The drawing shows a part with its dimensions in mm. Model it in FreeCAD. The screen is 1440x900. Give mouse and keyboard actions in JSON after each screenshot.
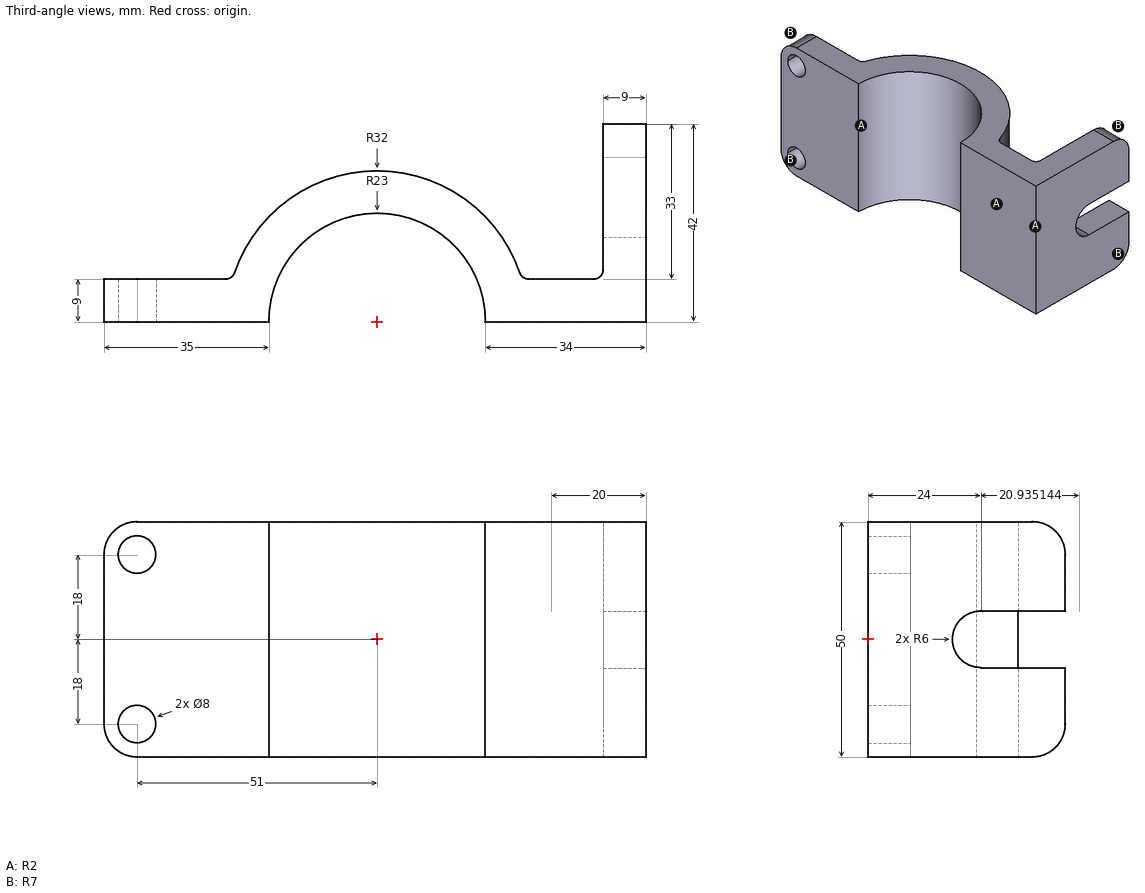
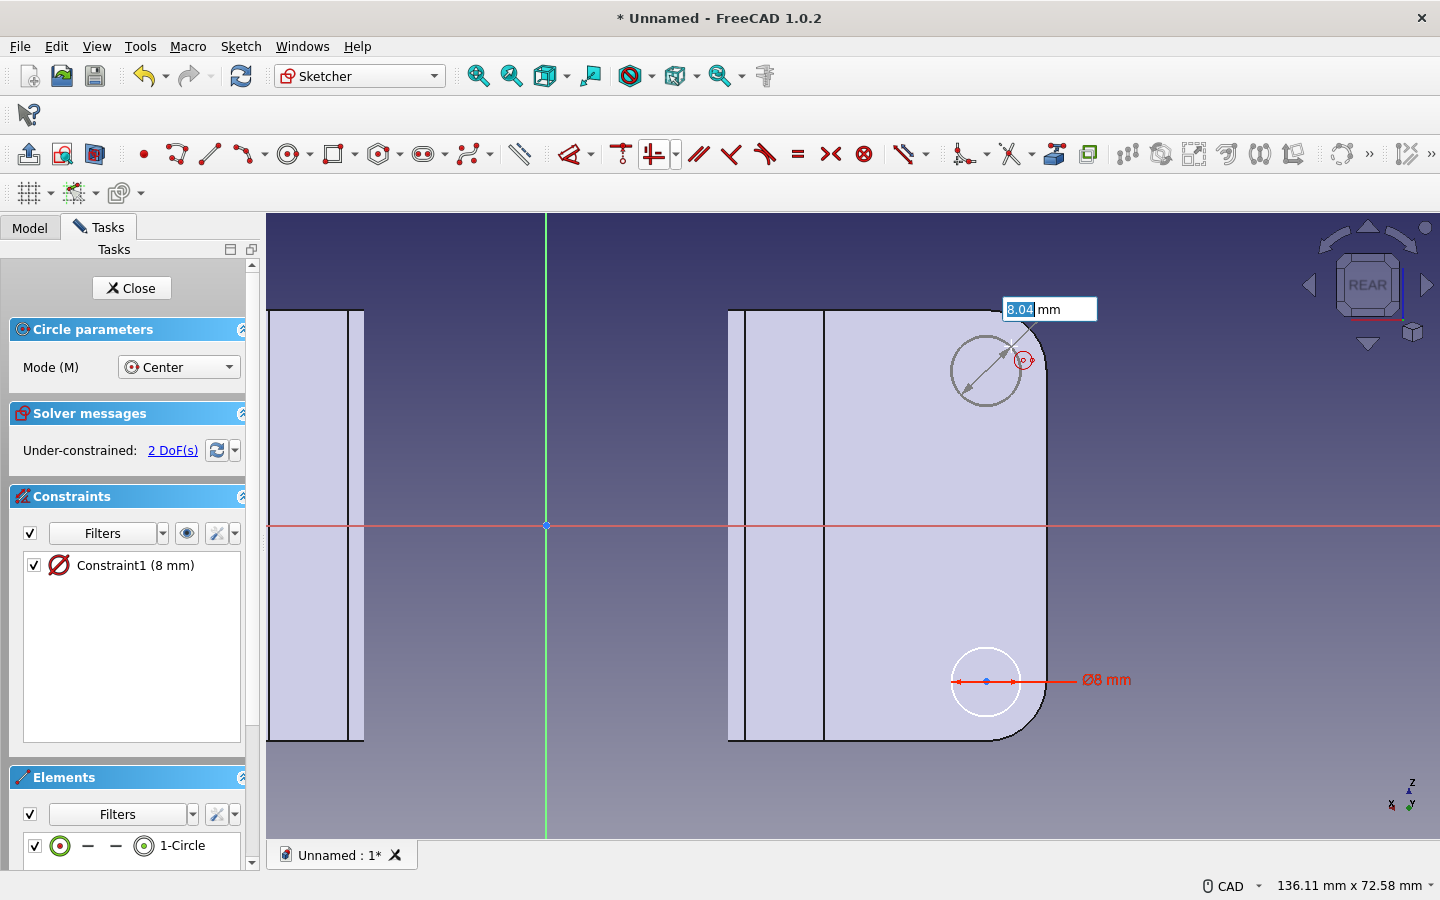
{"action": "type", "text": "8"}
{"action": "key", "text": "Return"}
{"action": "key", "text": "Escape"}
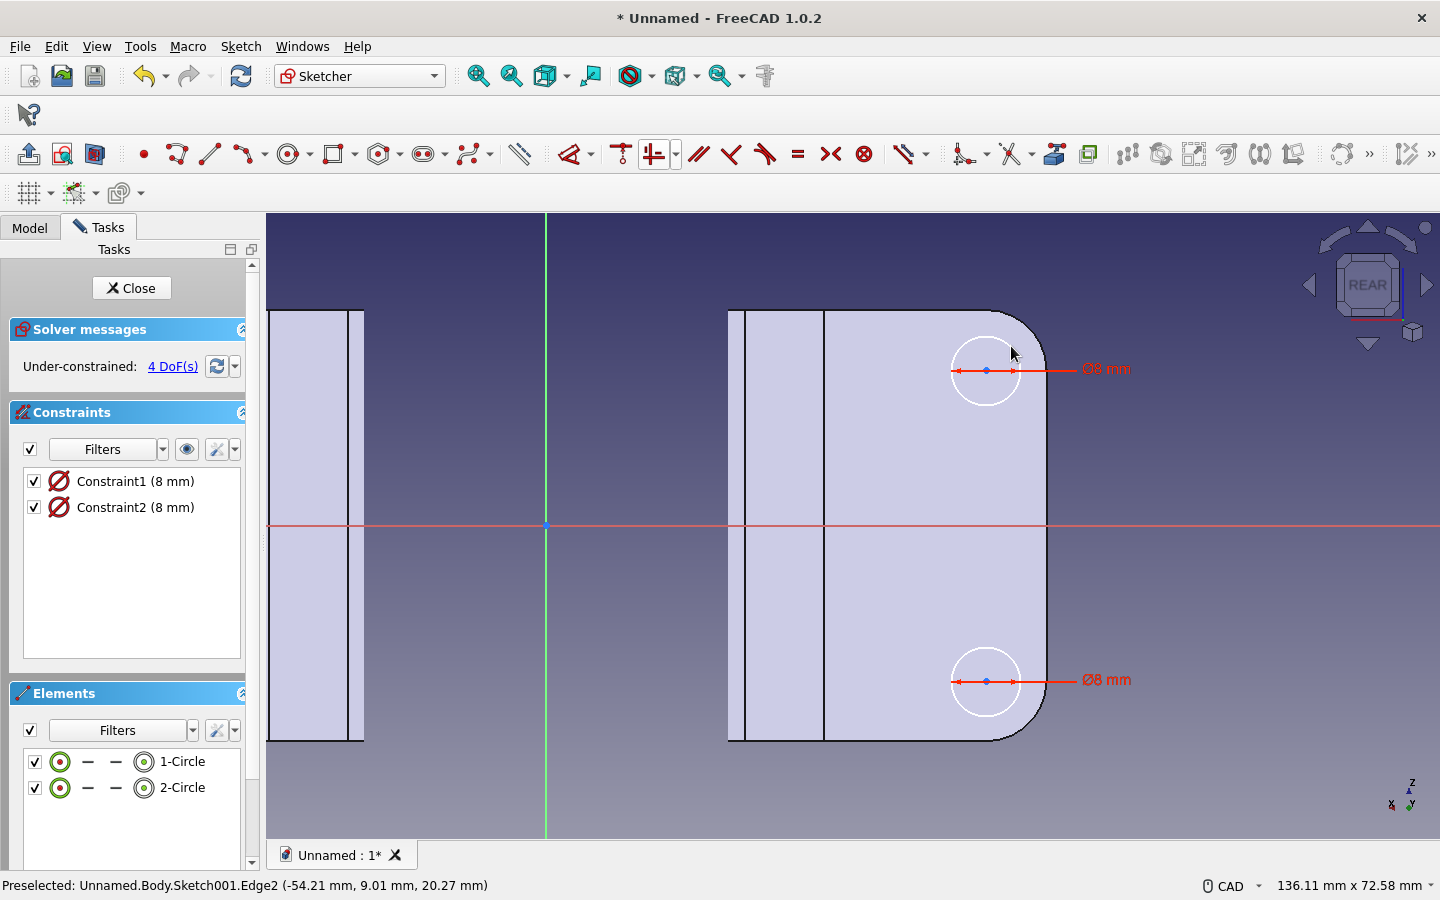
{"action": "left_click", "coordinate": [986, 682]}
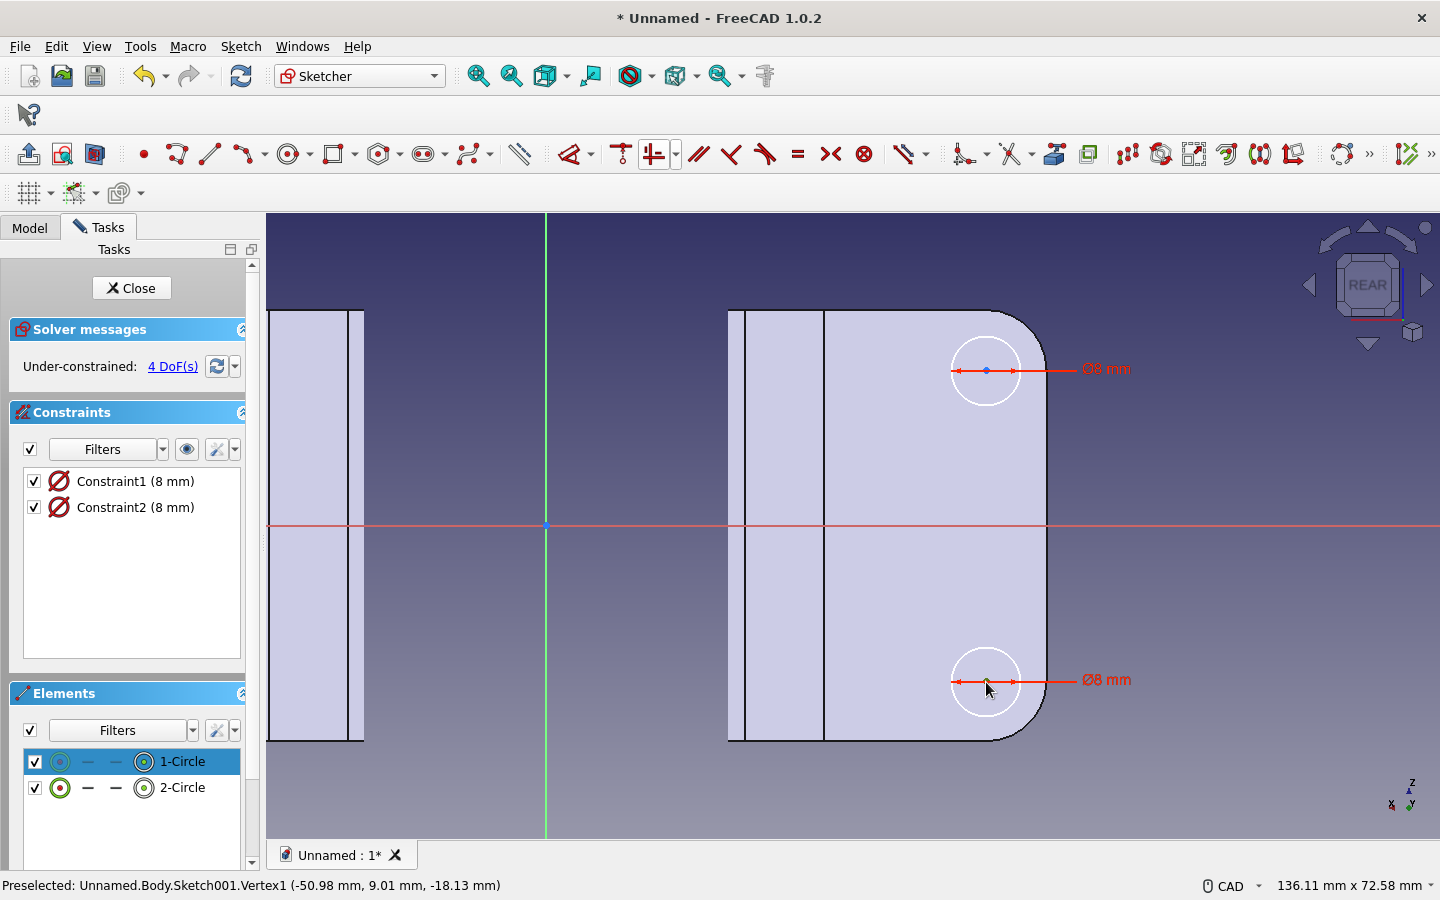
{"action": "left_click", "coordinate": [986, 371]}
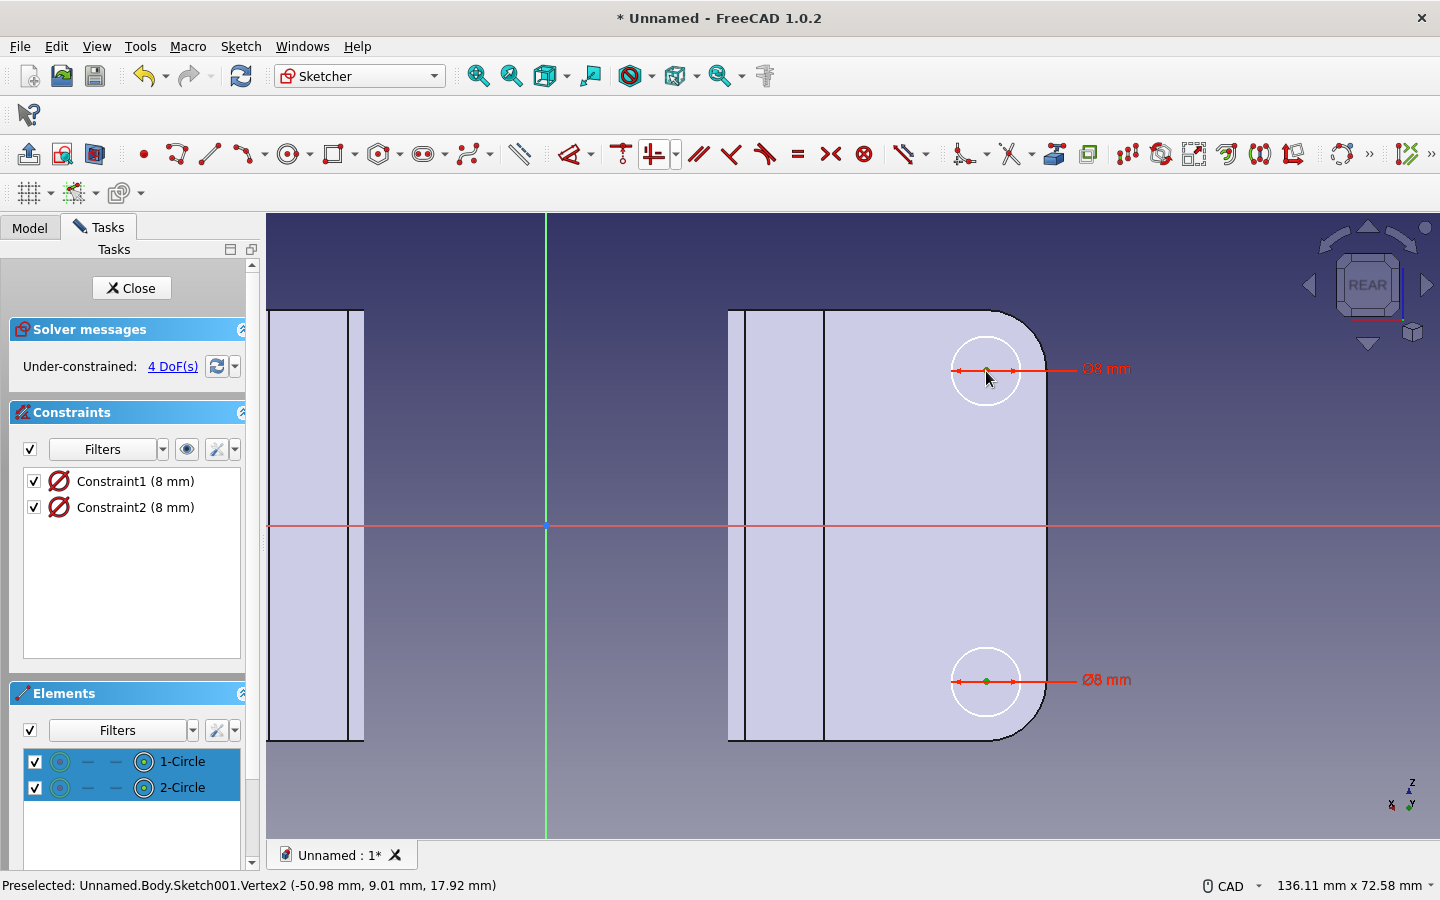
{"action": "key", "text": "v"}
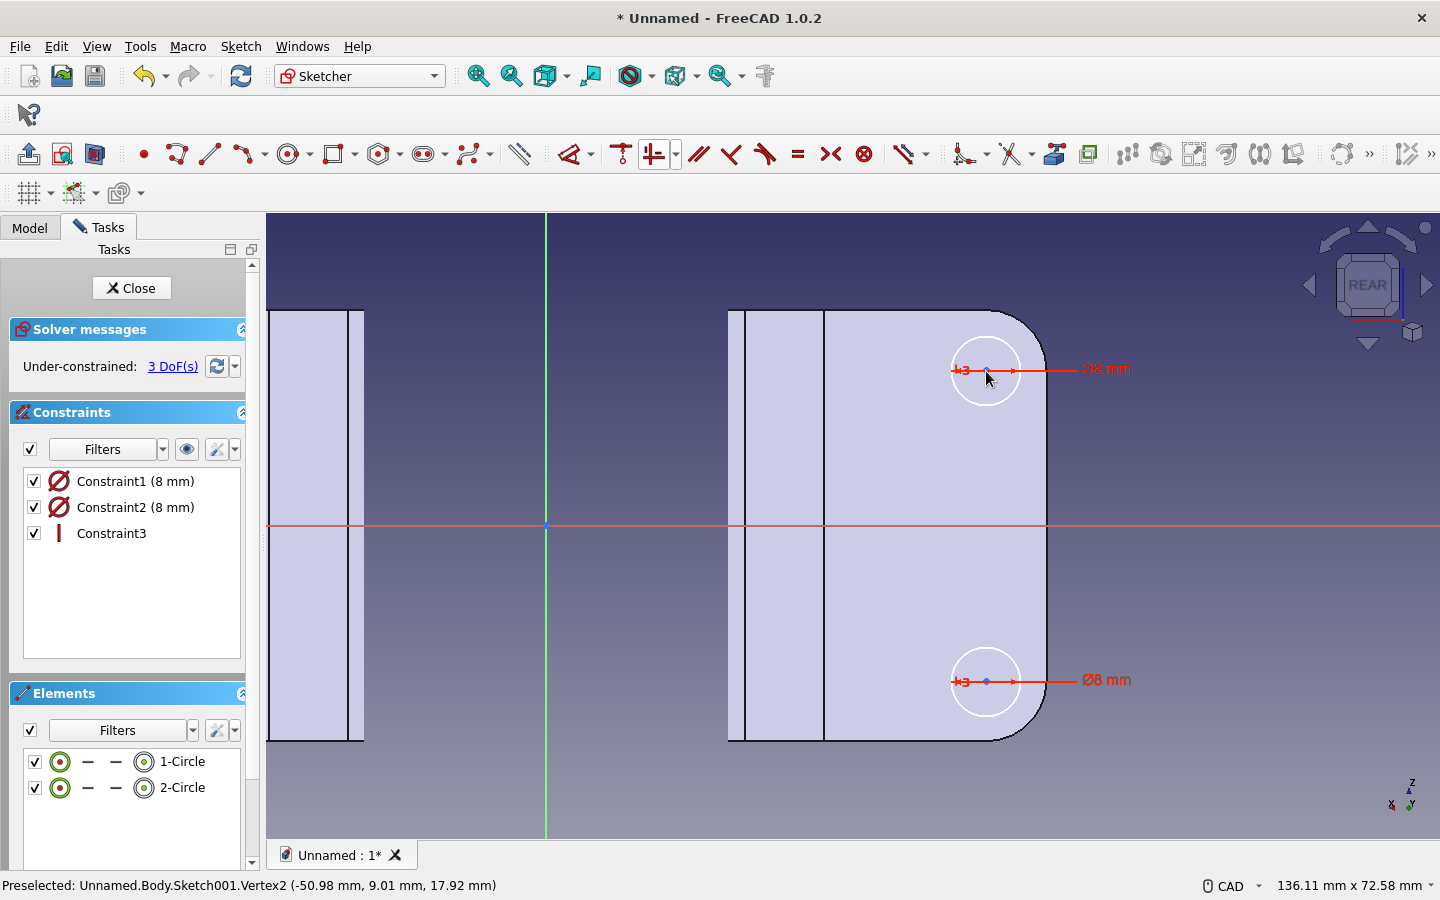
{"action": "left_click", "coordinate": [568, 154]}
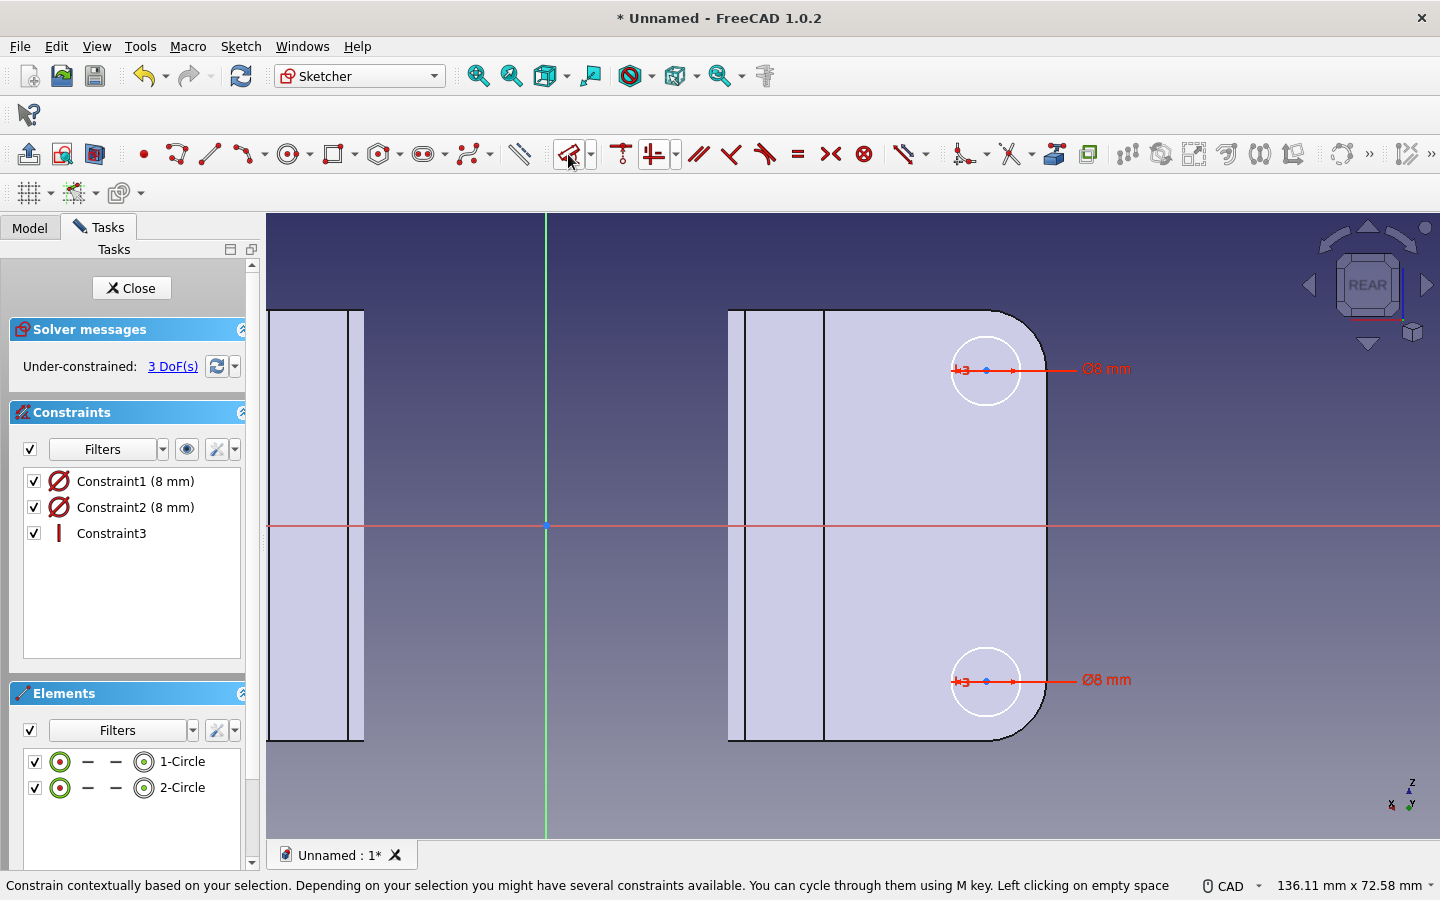
{"action": "left_click", "coordinate": [986, 682]}
{"action": "left_click", "coordinate": [766, 716]}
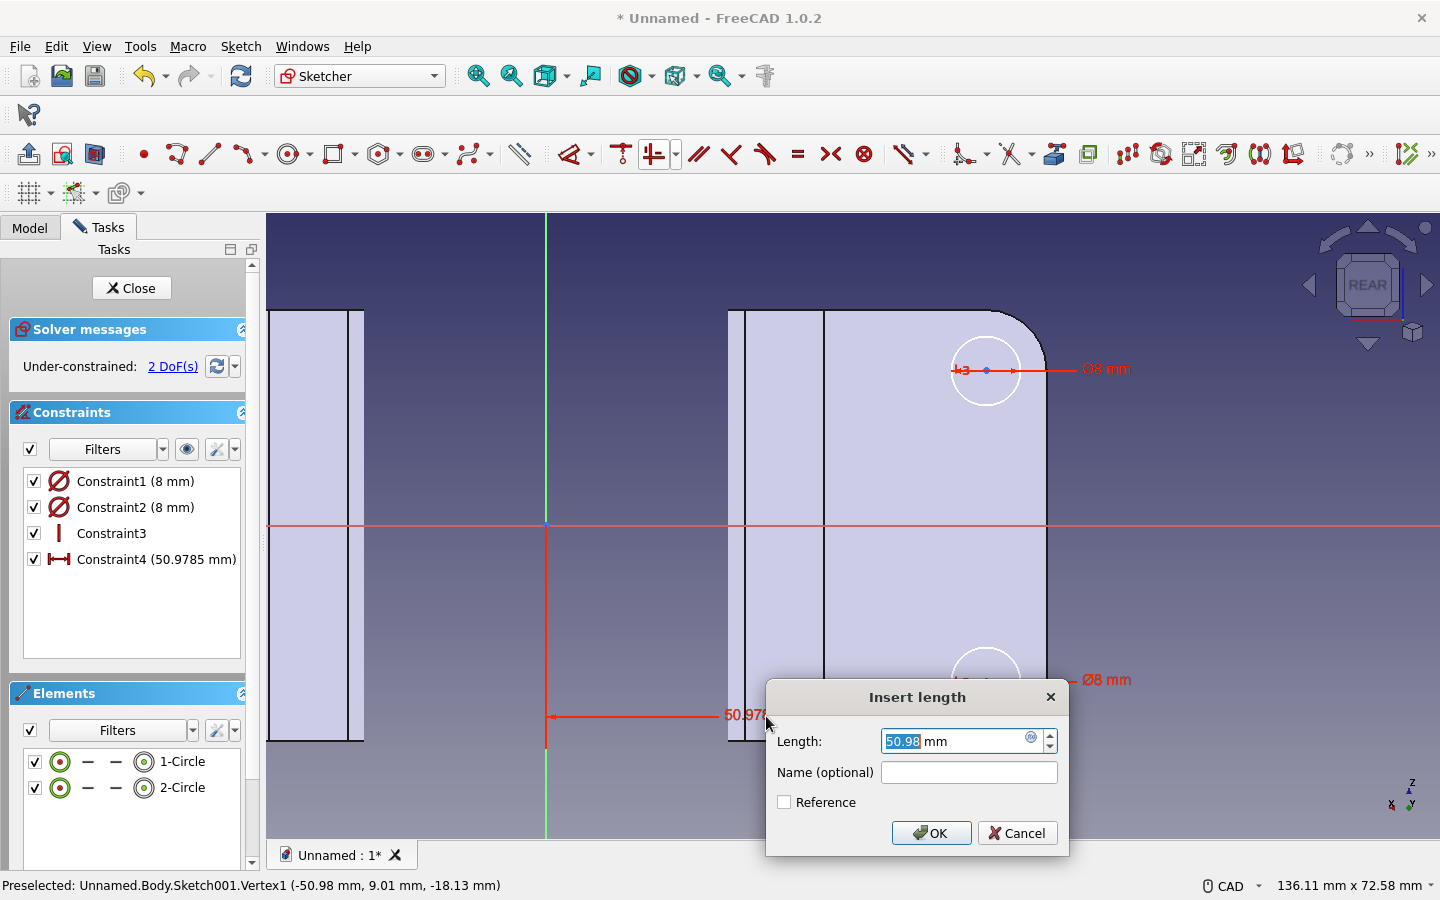
{"action": "type", "text": "51"}
{"action": "key", "text": "Return"}